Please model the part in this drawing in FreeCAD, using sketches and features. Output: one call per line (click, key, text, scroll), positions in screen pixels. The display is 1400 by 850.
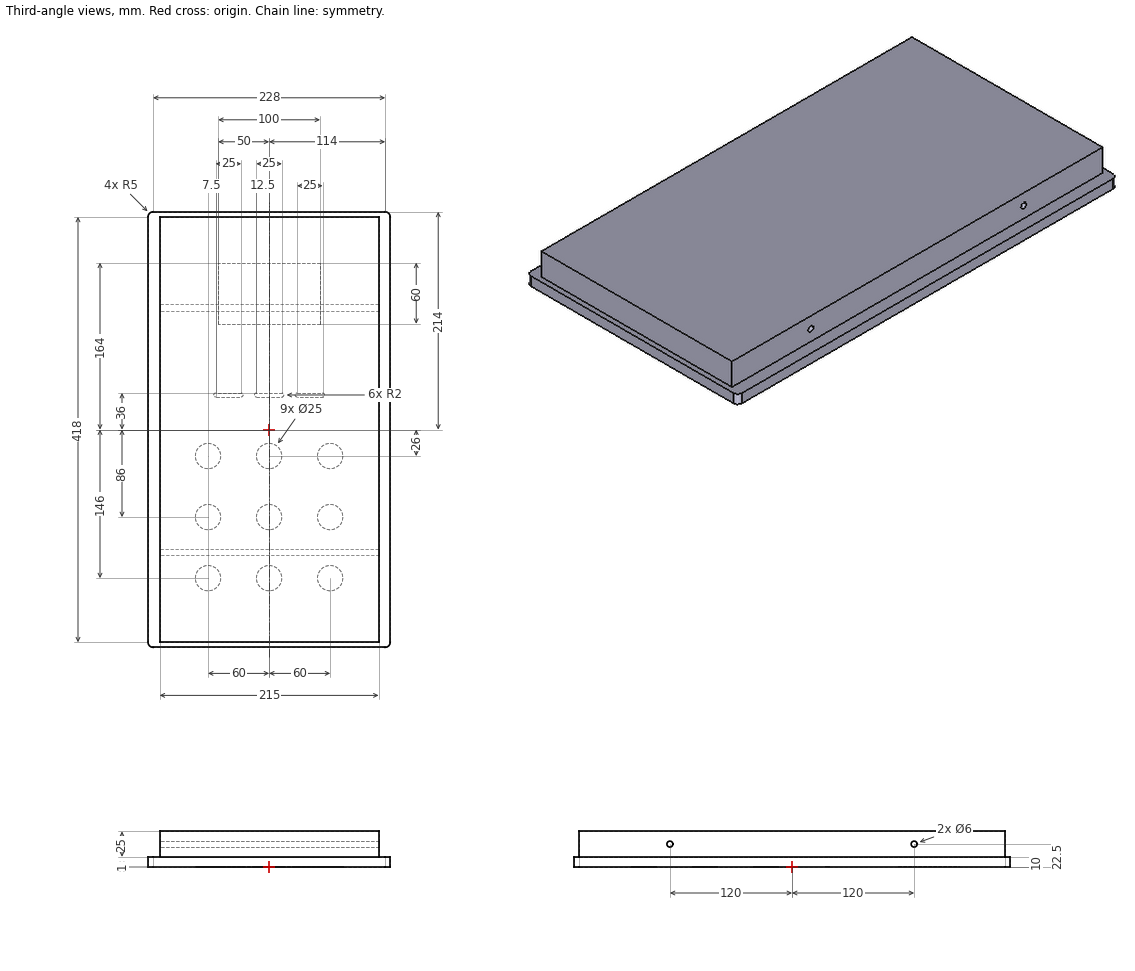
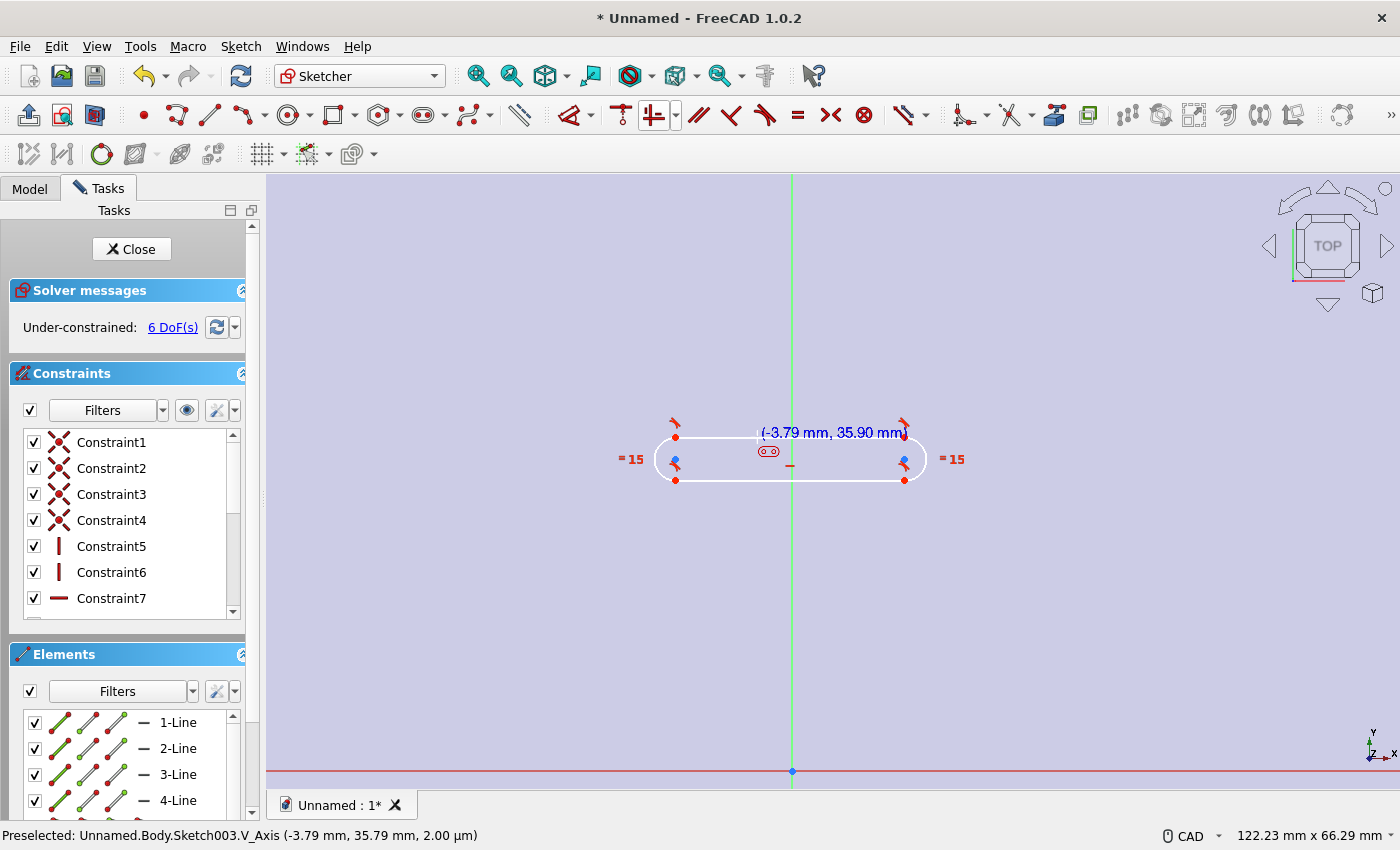
scroll(305, 456, up, 2)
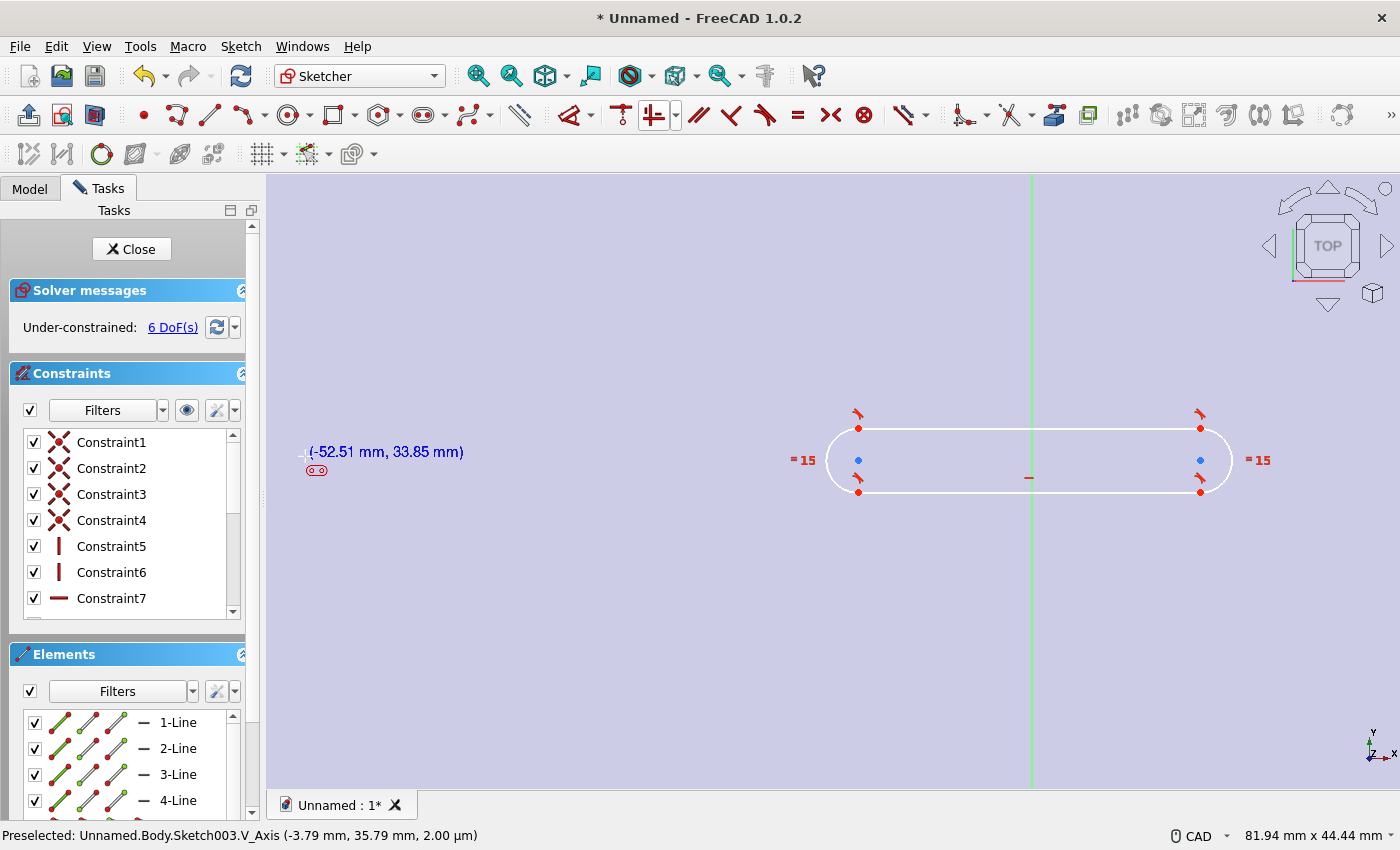
scroll(738, 441, down, 12)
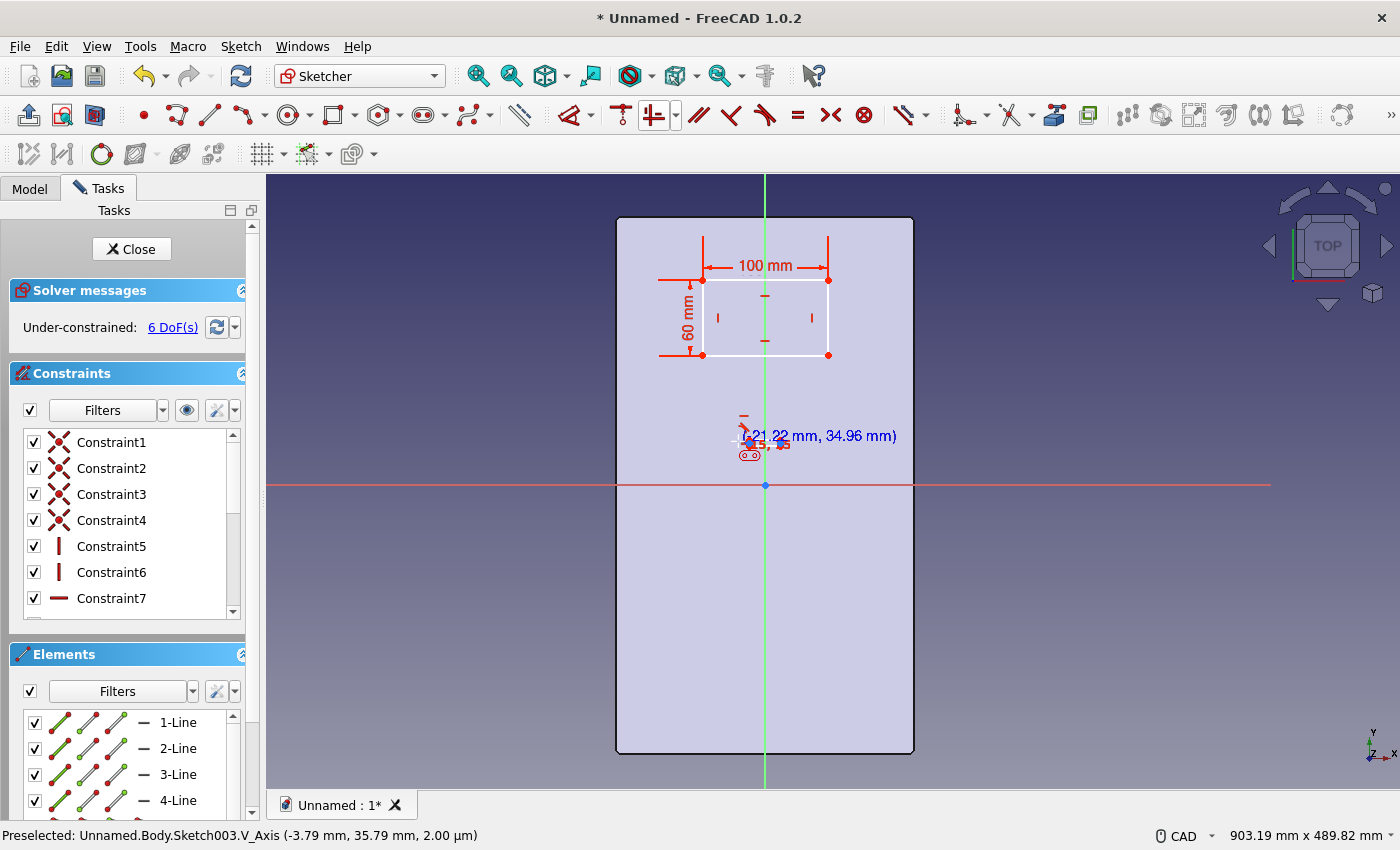
click(699, 443)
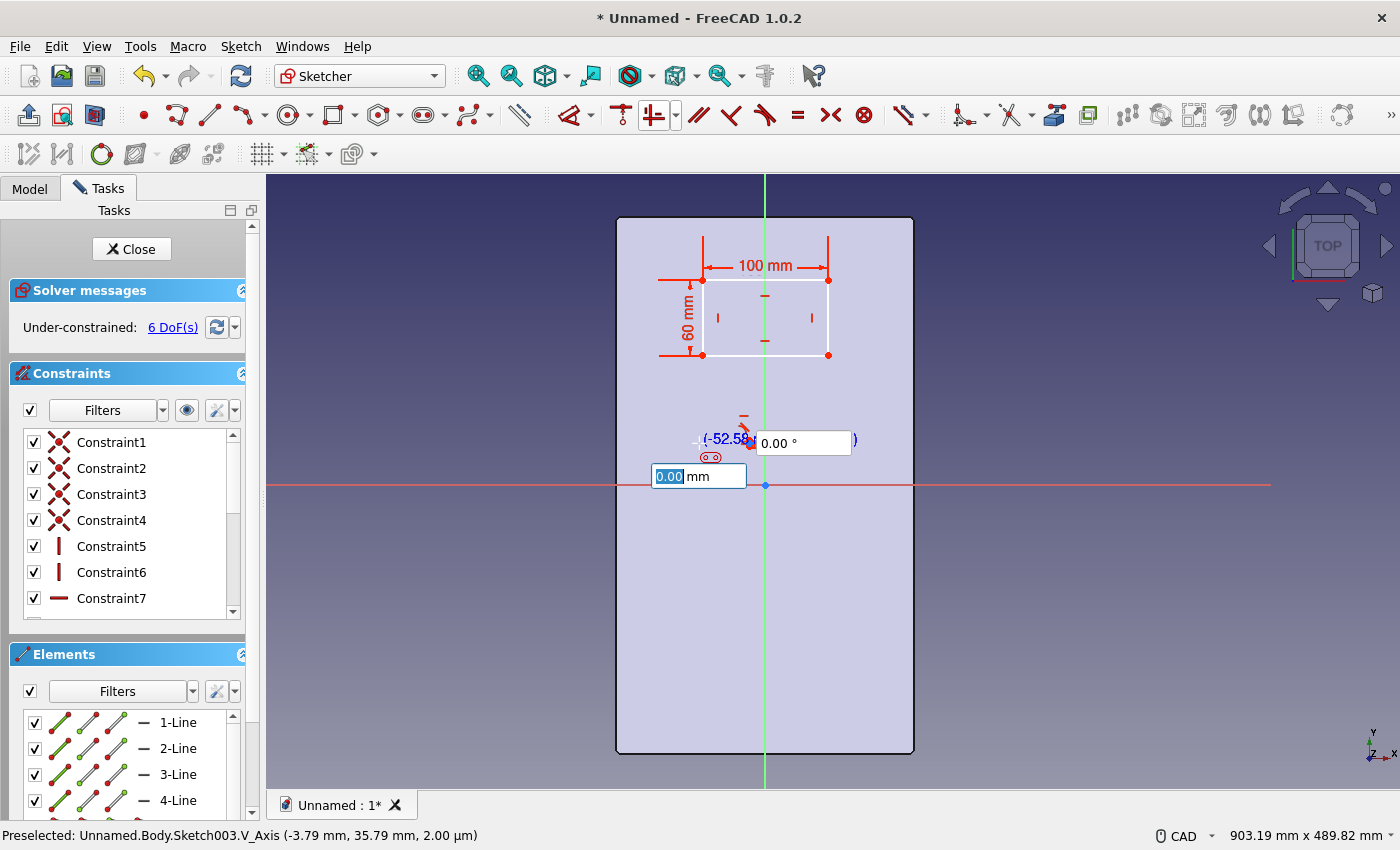
click(730, 443)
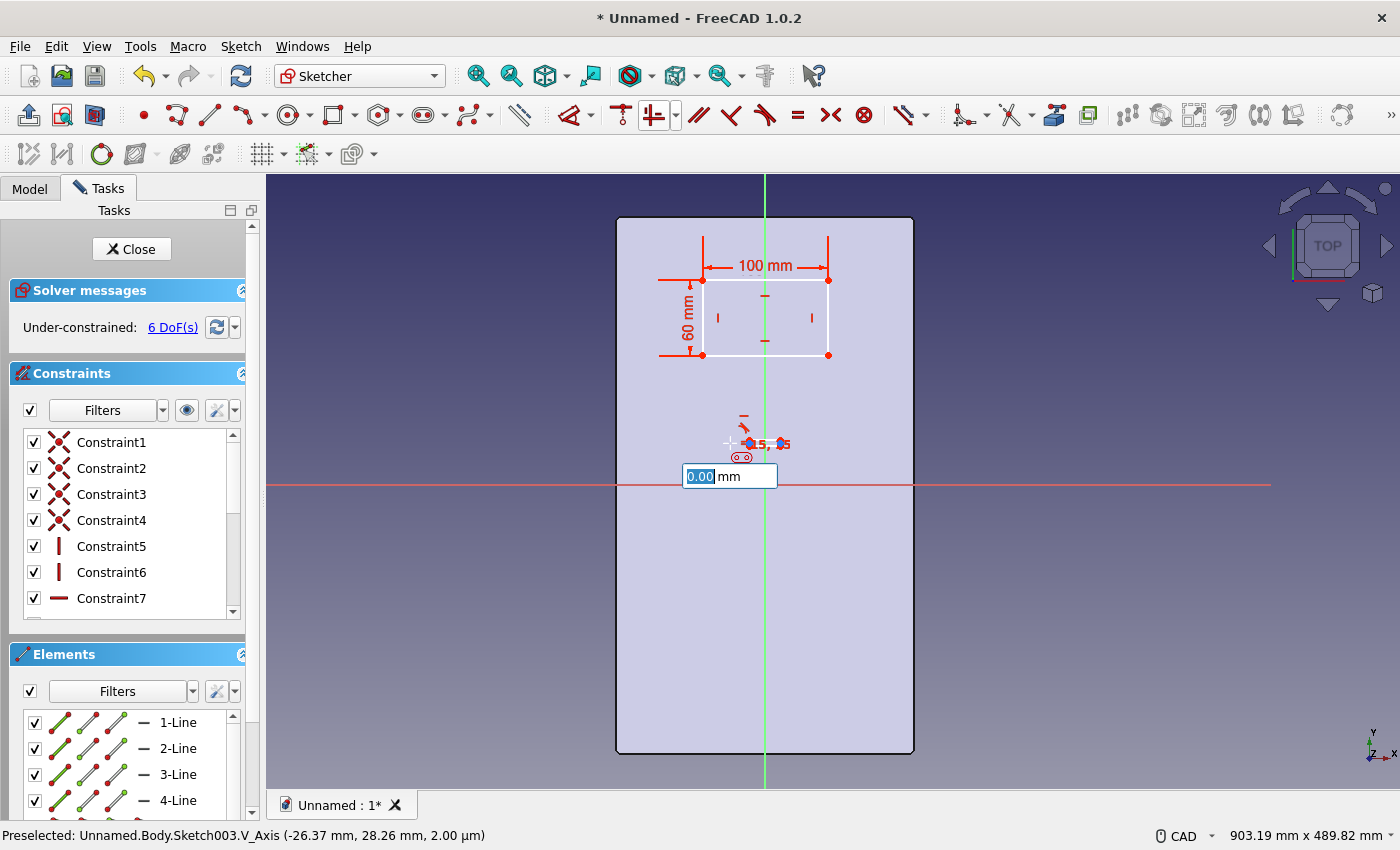
scroll(715, 440, up, 10)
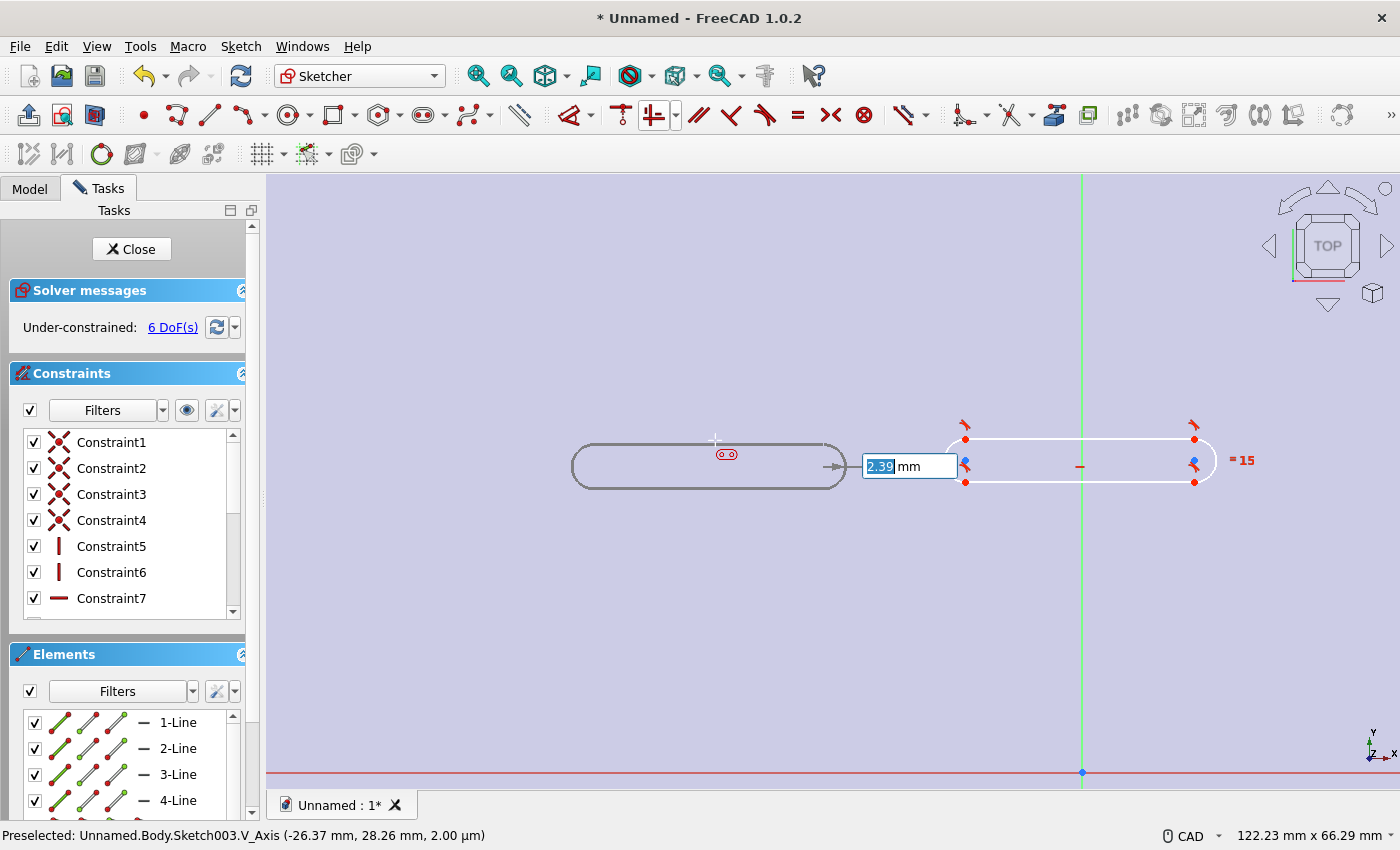
click(711, 439)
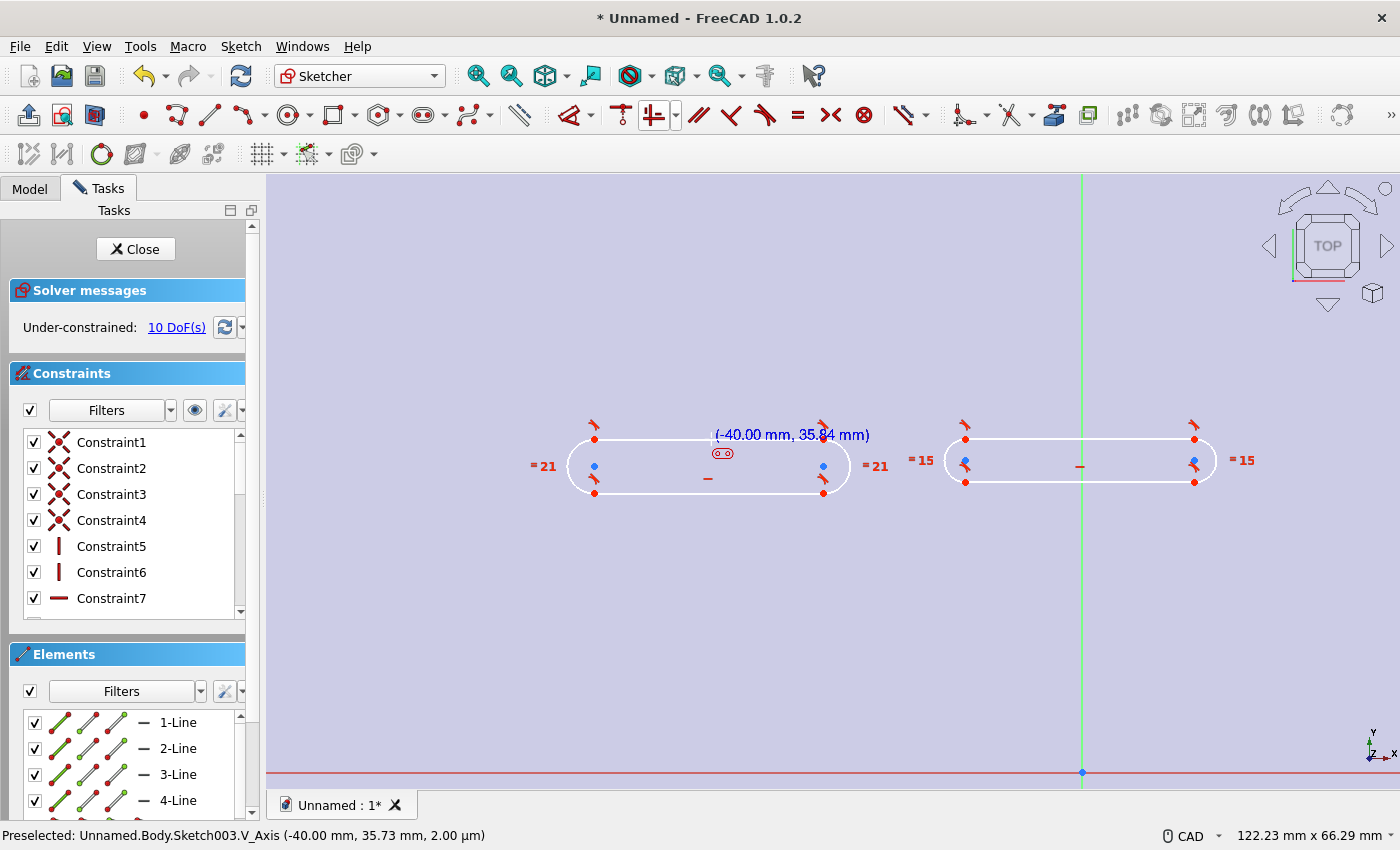
scroll(715, 440, down, 10)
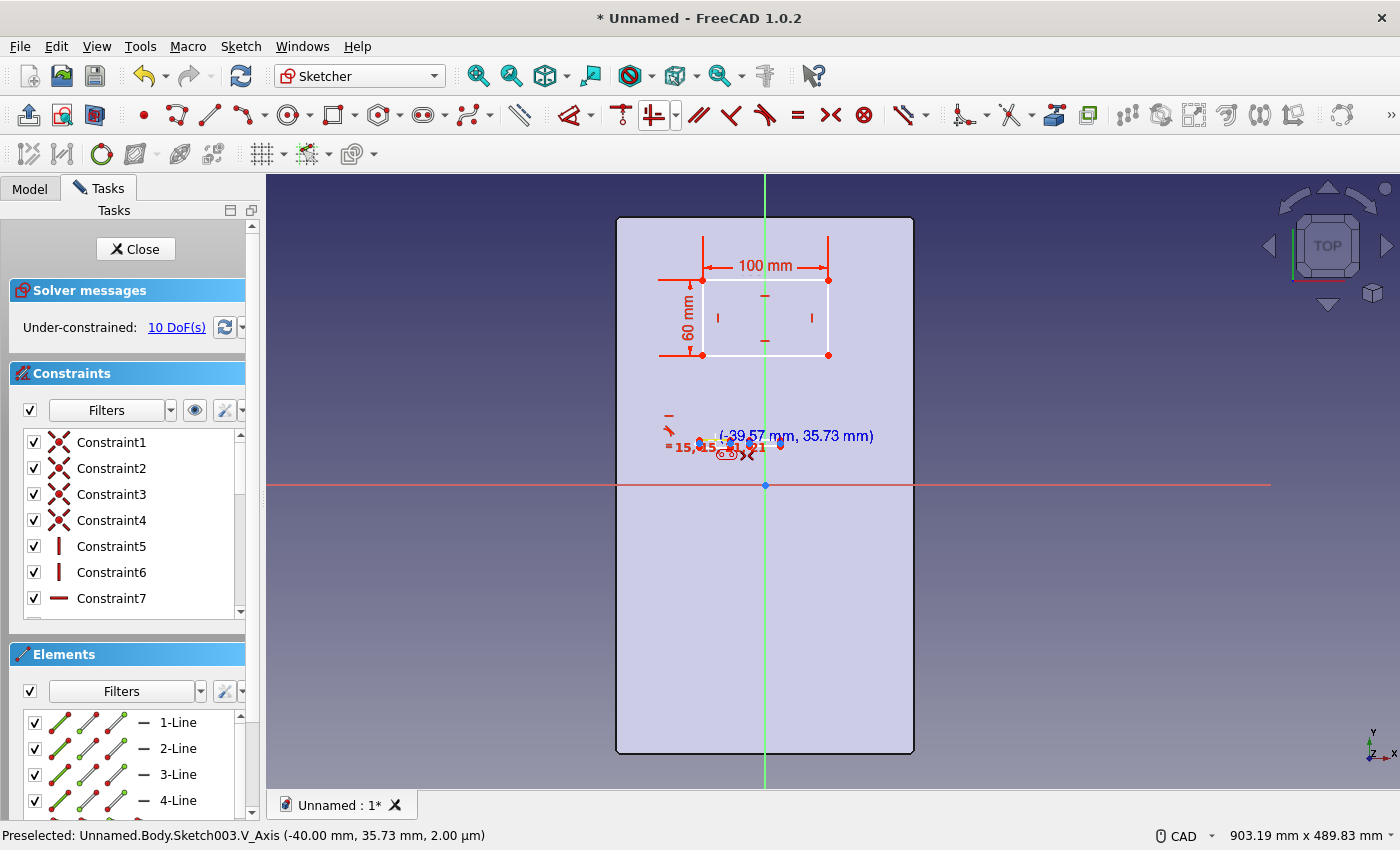
scroll(800, 443, up, 12)